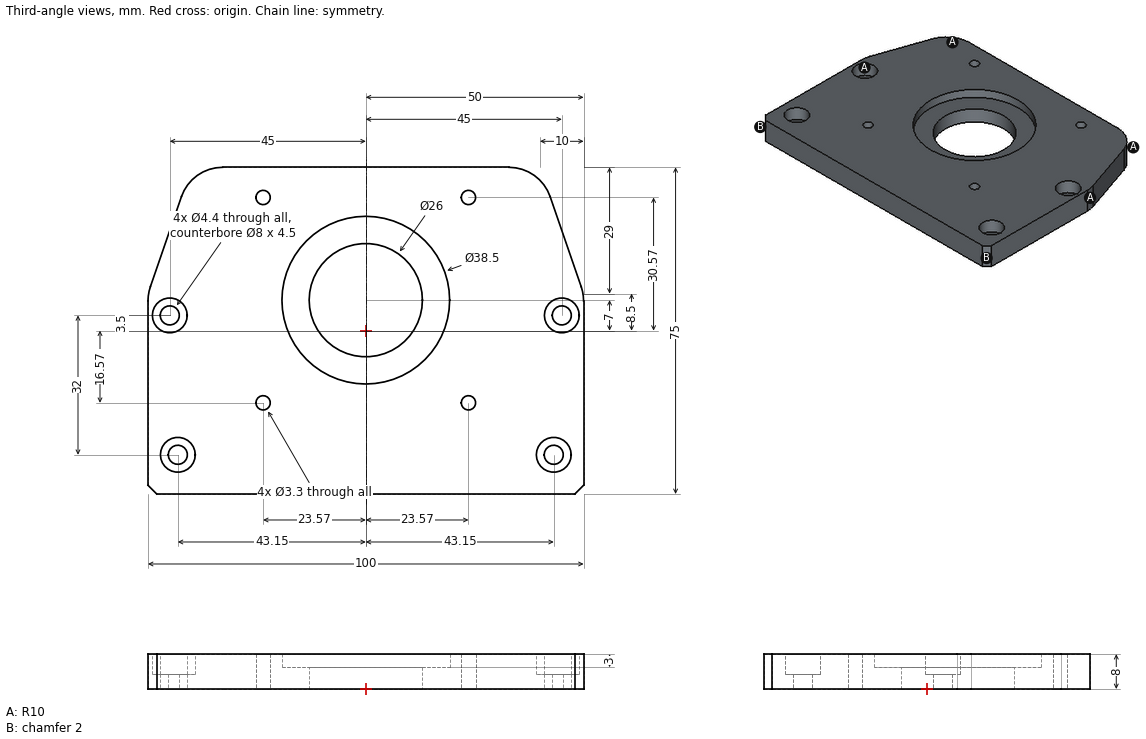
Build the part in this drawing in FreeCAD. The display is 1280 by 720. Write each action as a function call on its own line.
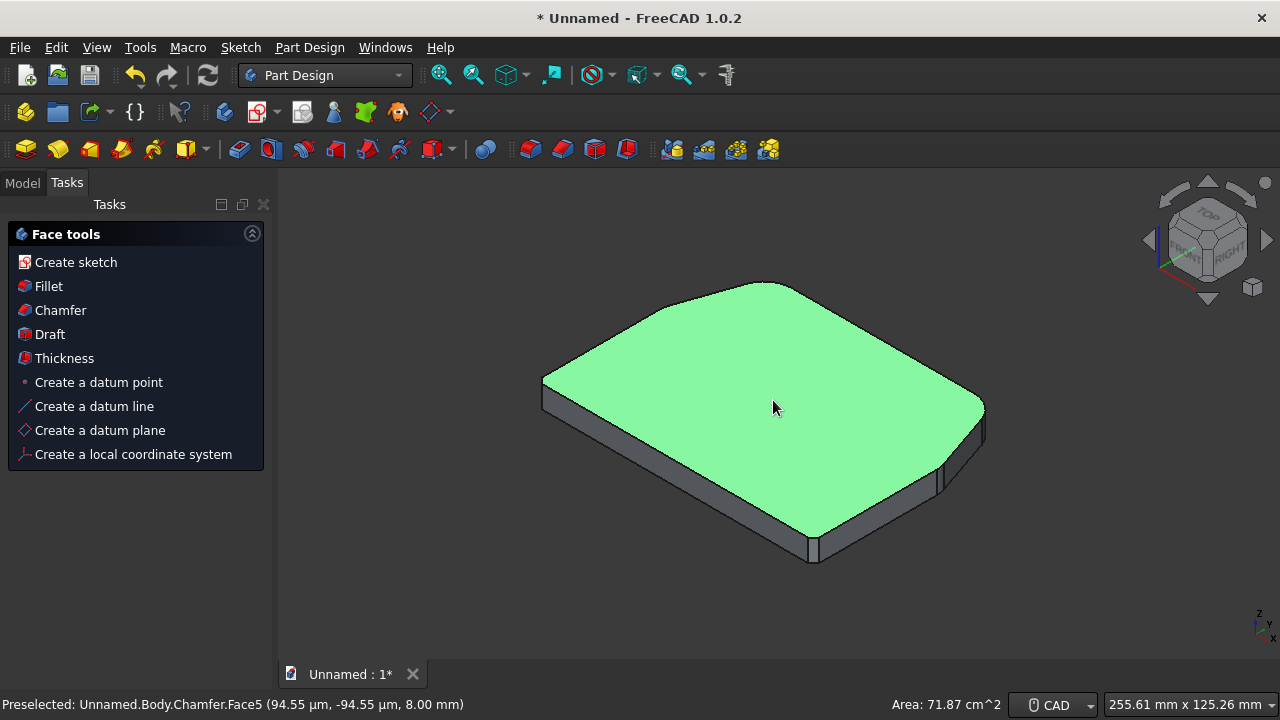
click(258, 112)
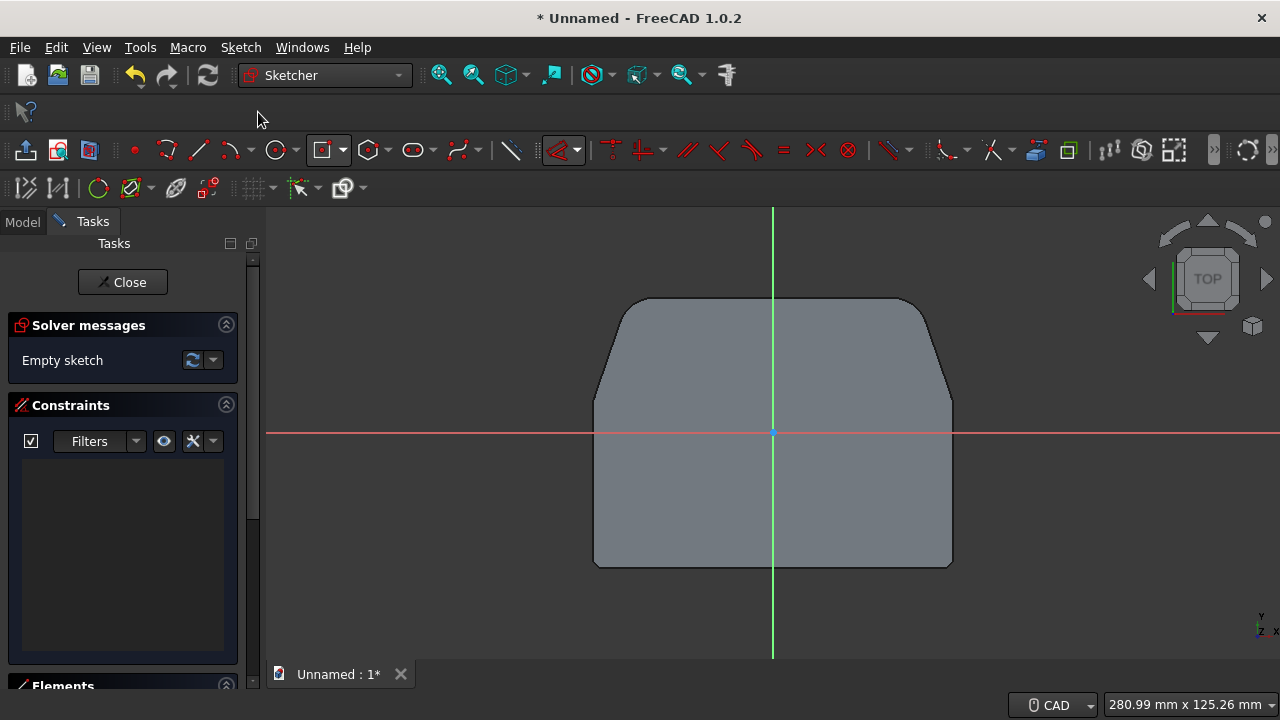
scroll(856, 377, up, 3)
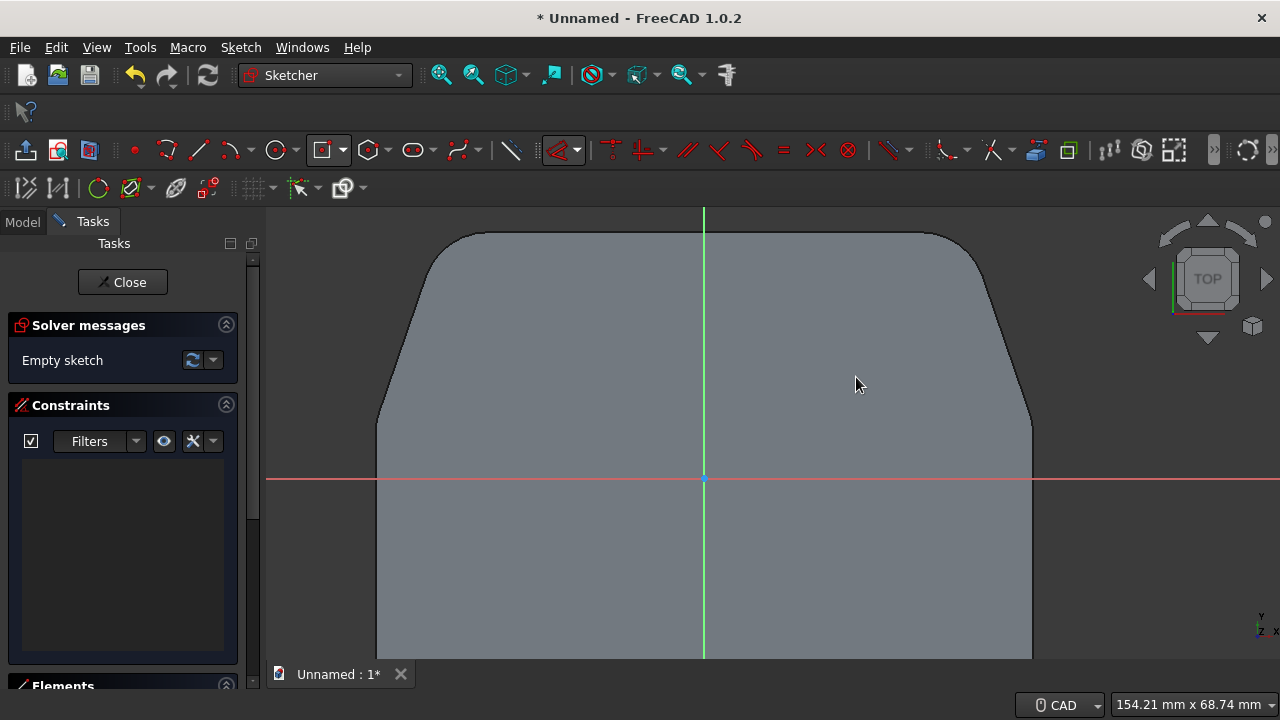
click(276, 150)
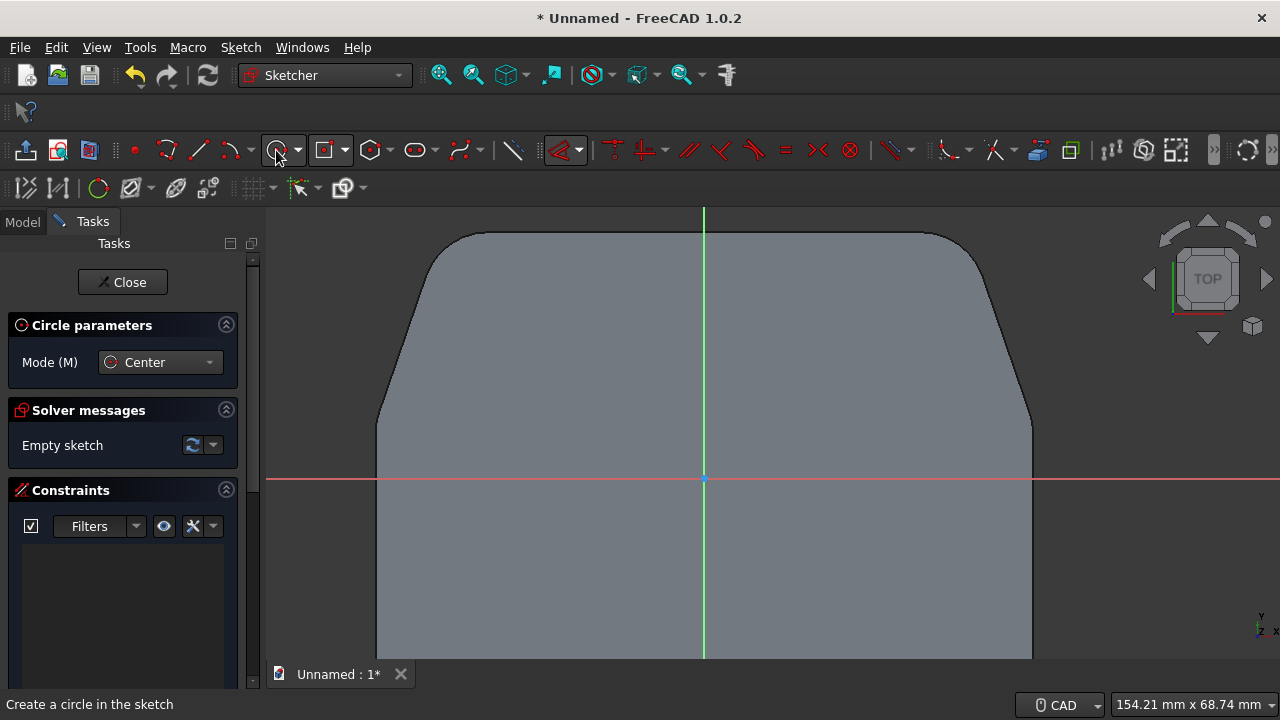
click(704, 433)
click(794, 343)
key(Escape)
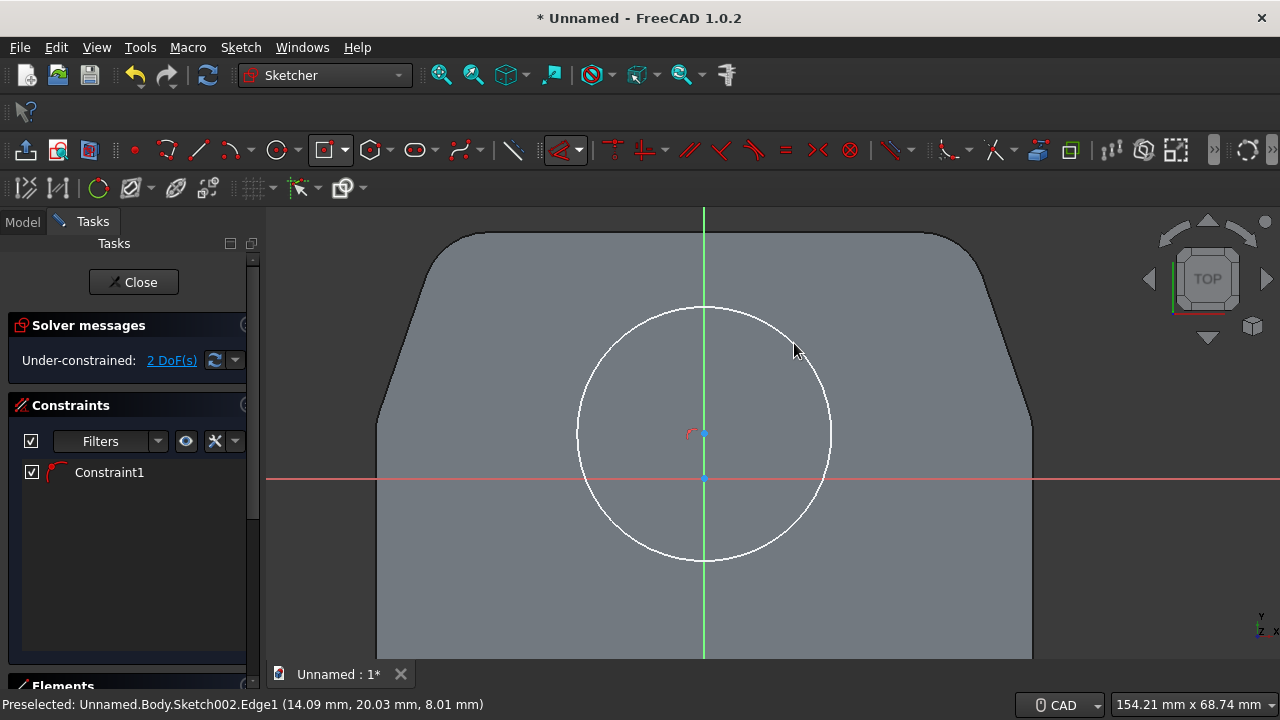
click(794, 344)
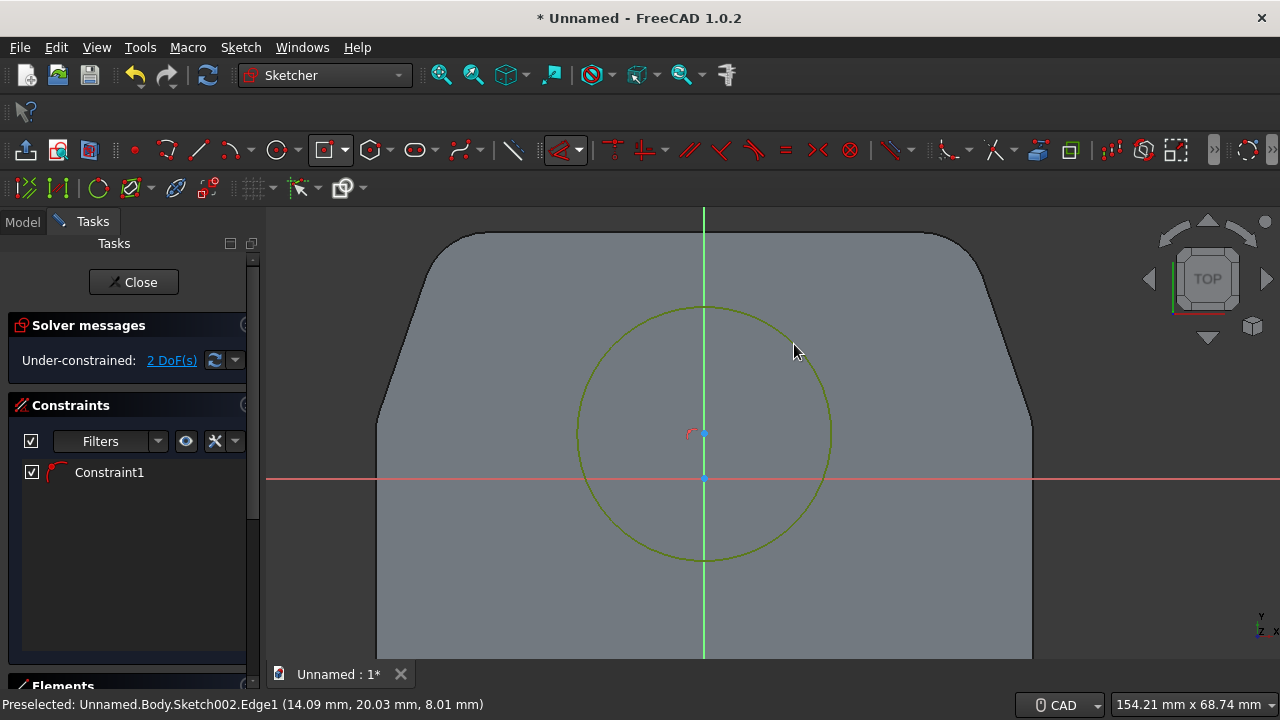
key(k)
key(o)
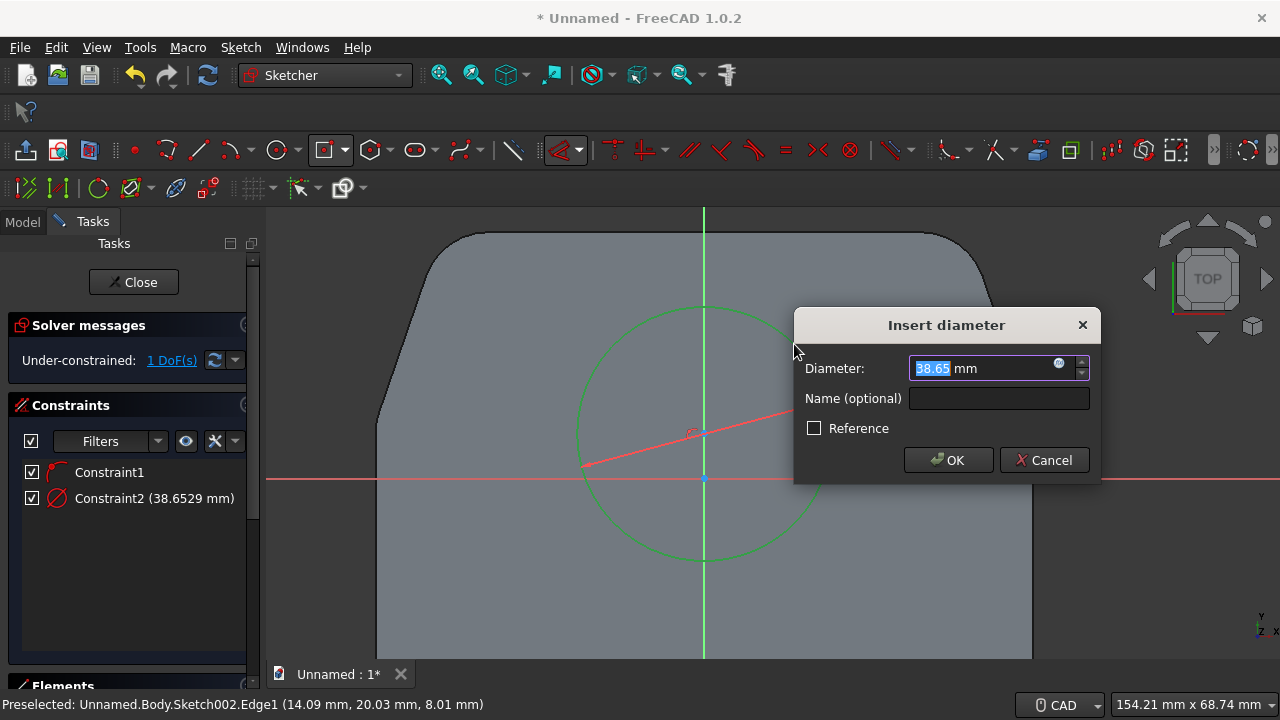
text(38.5)
key(Return)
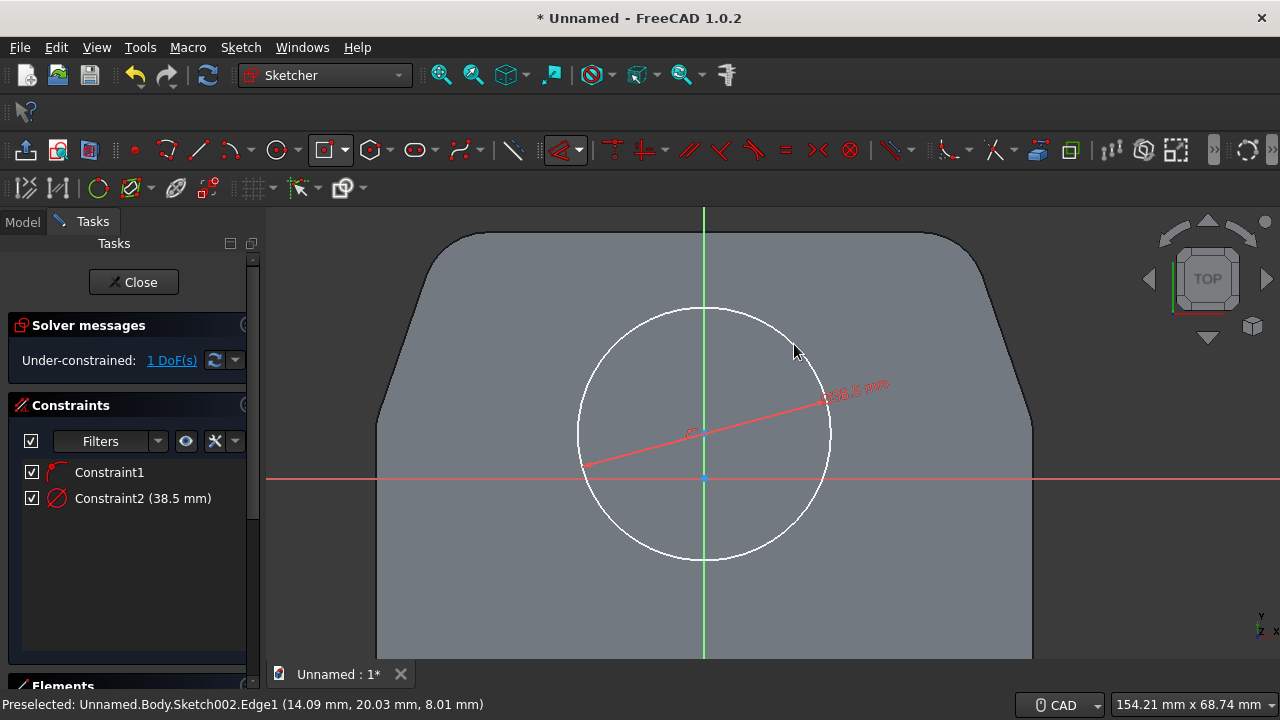
click(704, 434)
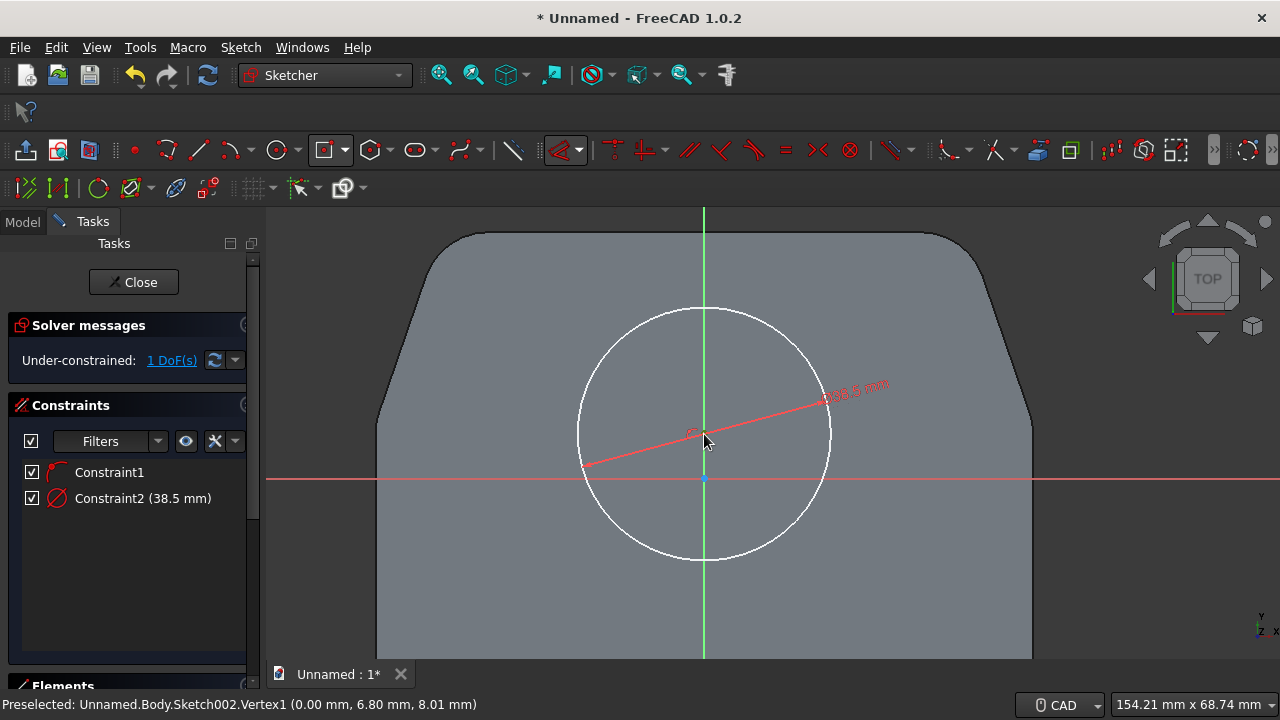
key(i)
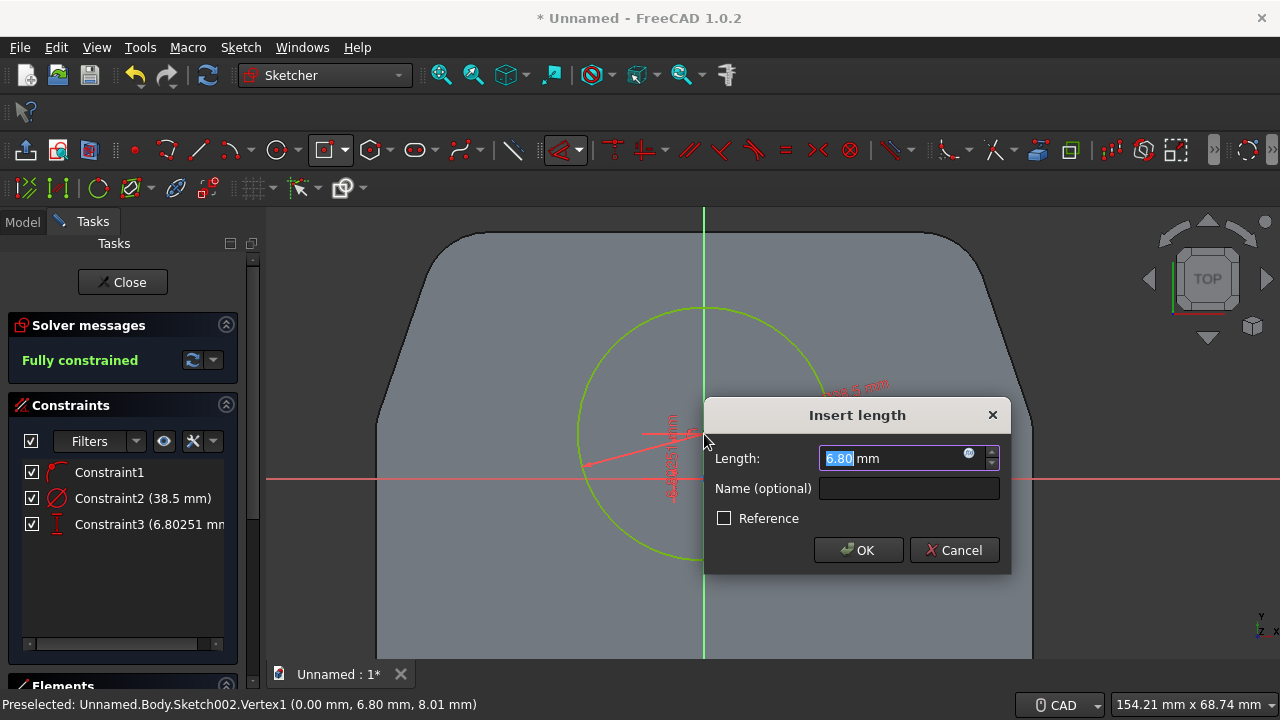
text(7)
key(Return)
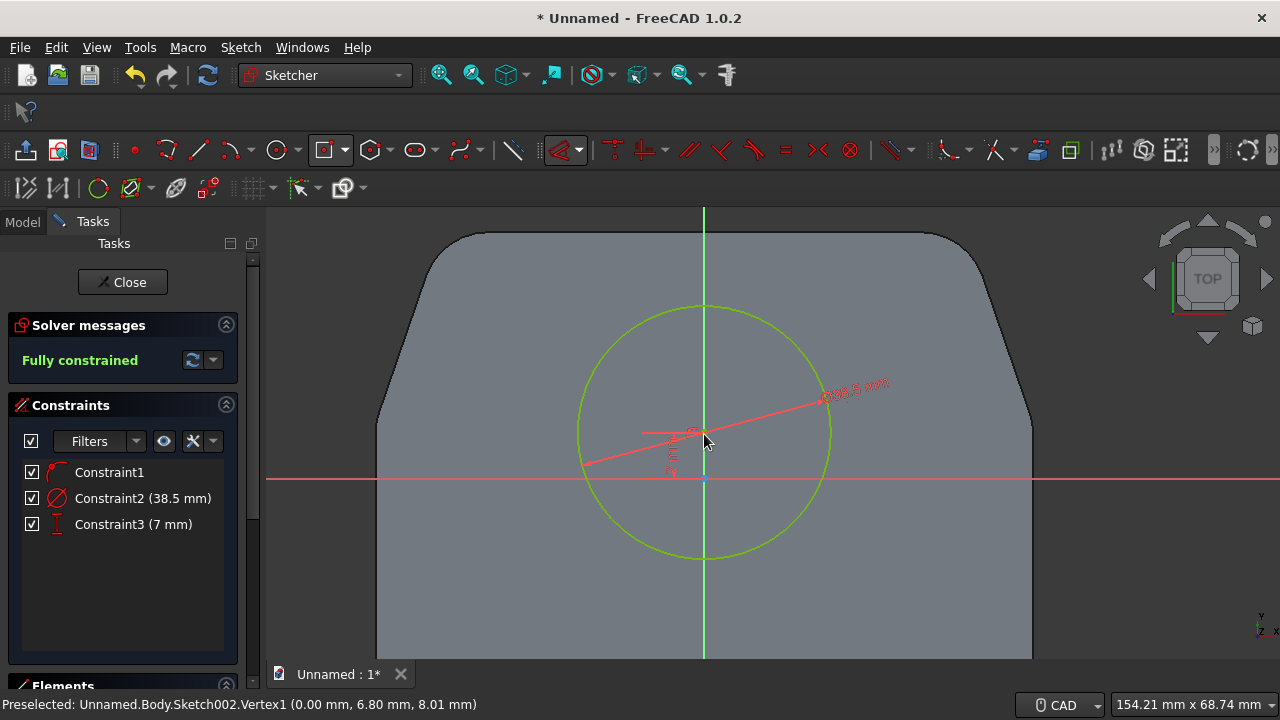
click(123, 282)